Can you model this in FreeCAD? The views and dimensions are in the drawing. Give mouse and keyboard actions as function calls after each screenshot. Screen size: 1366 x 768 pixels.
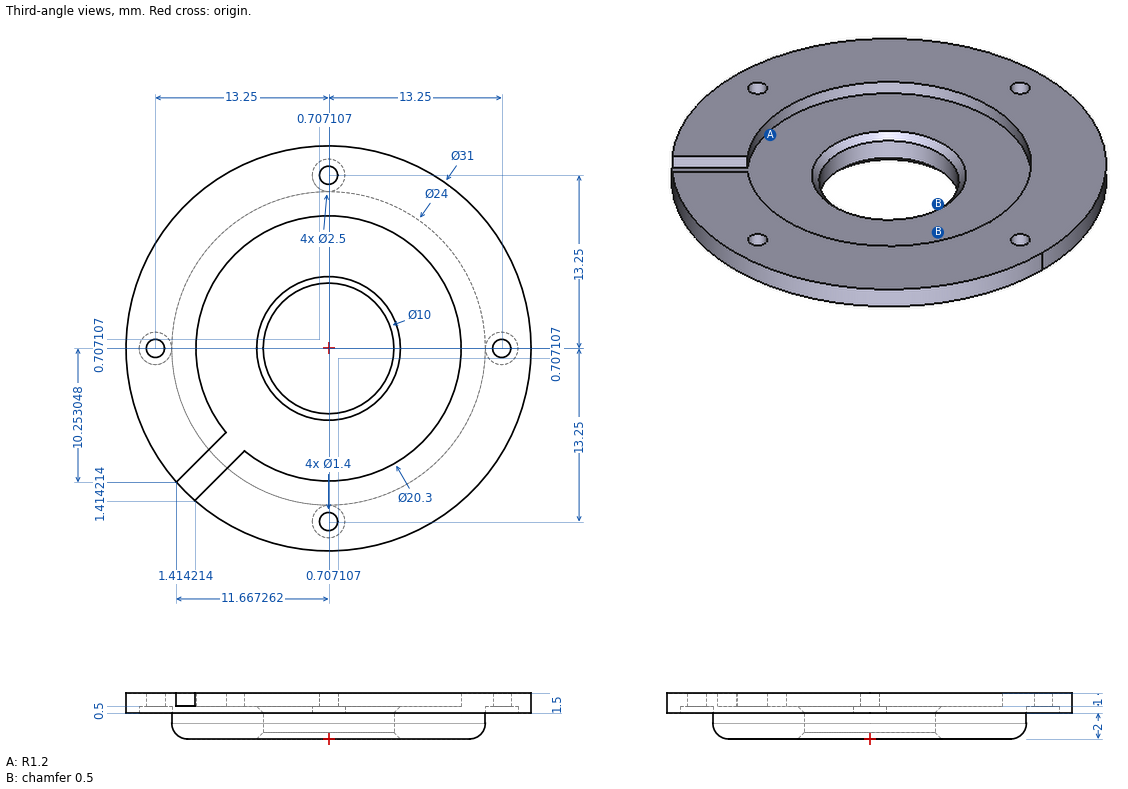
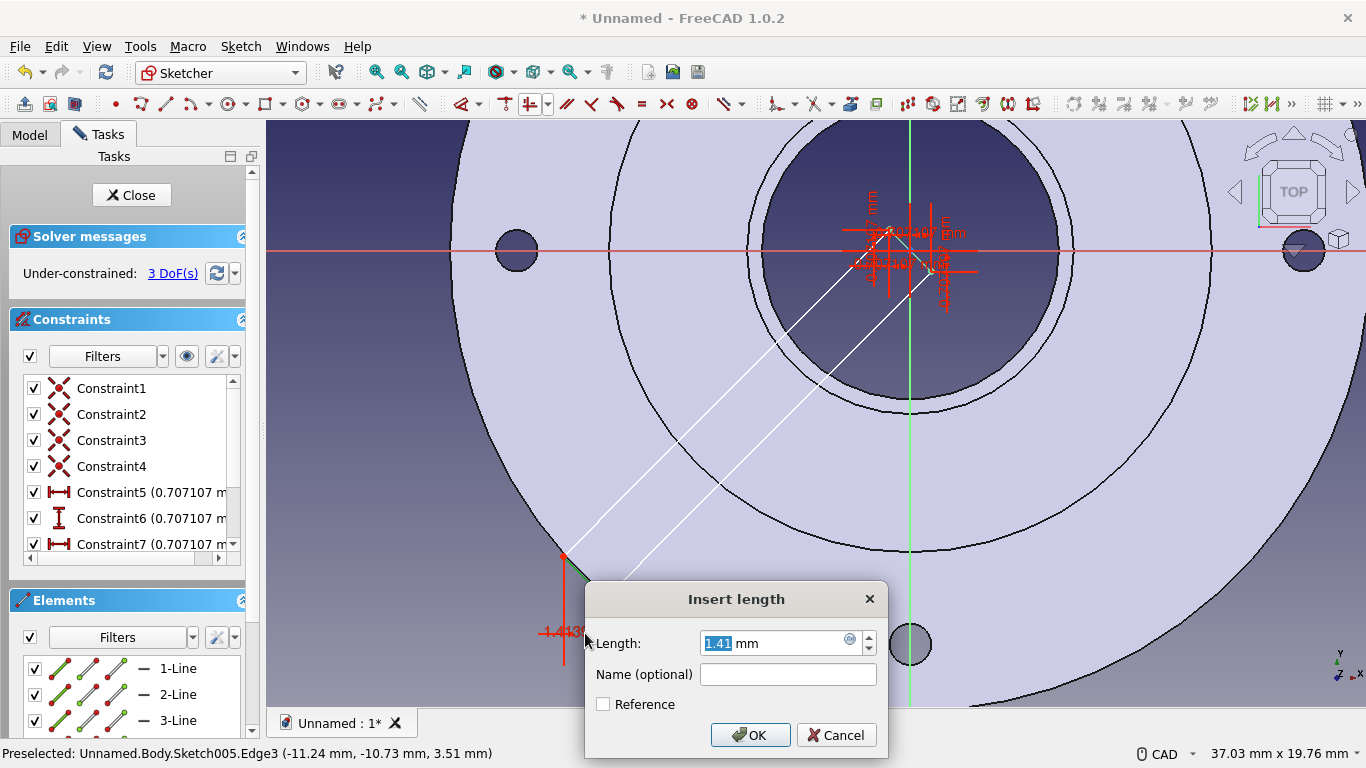
text(1.414214)
key(Return)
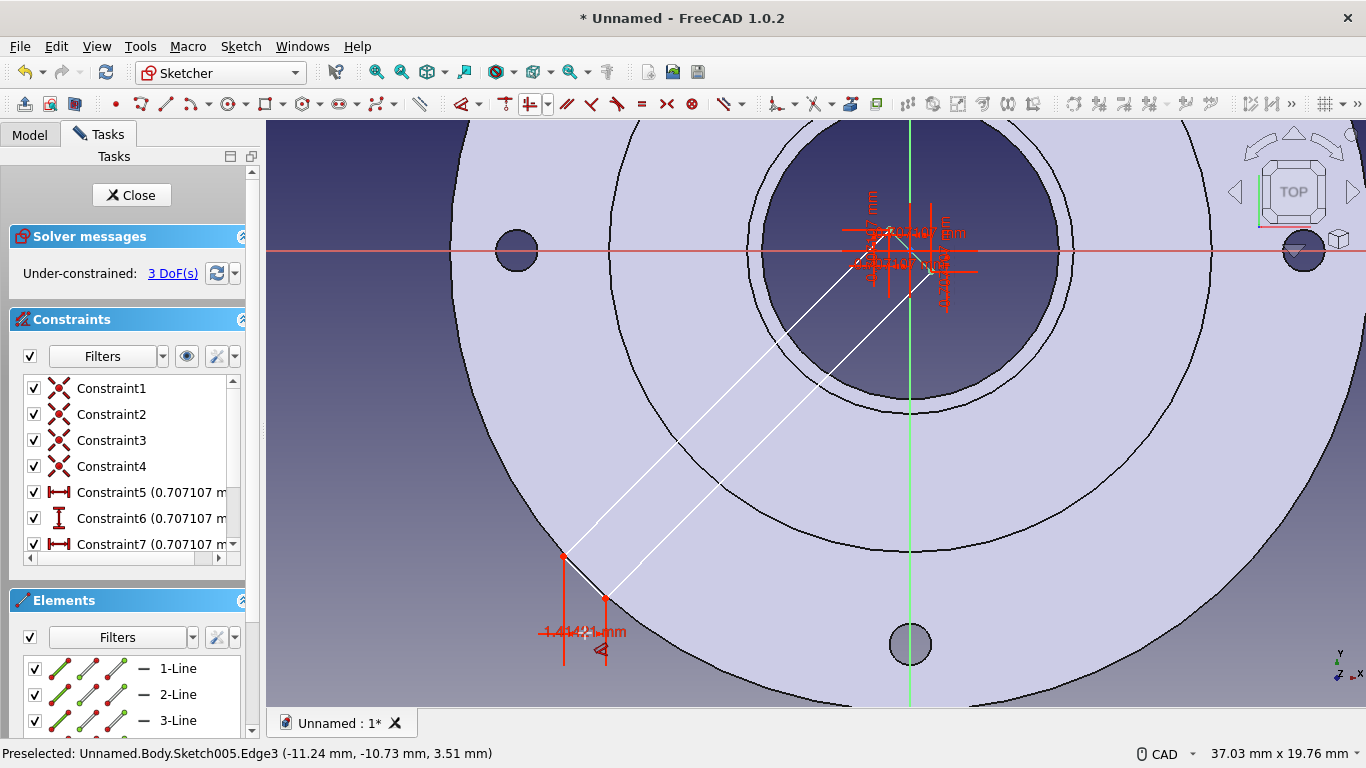
click(576, 569)
click(530, 578)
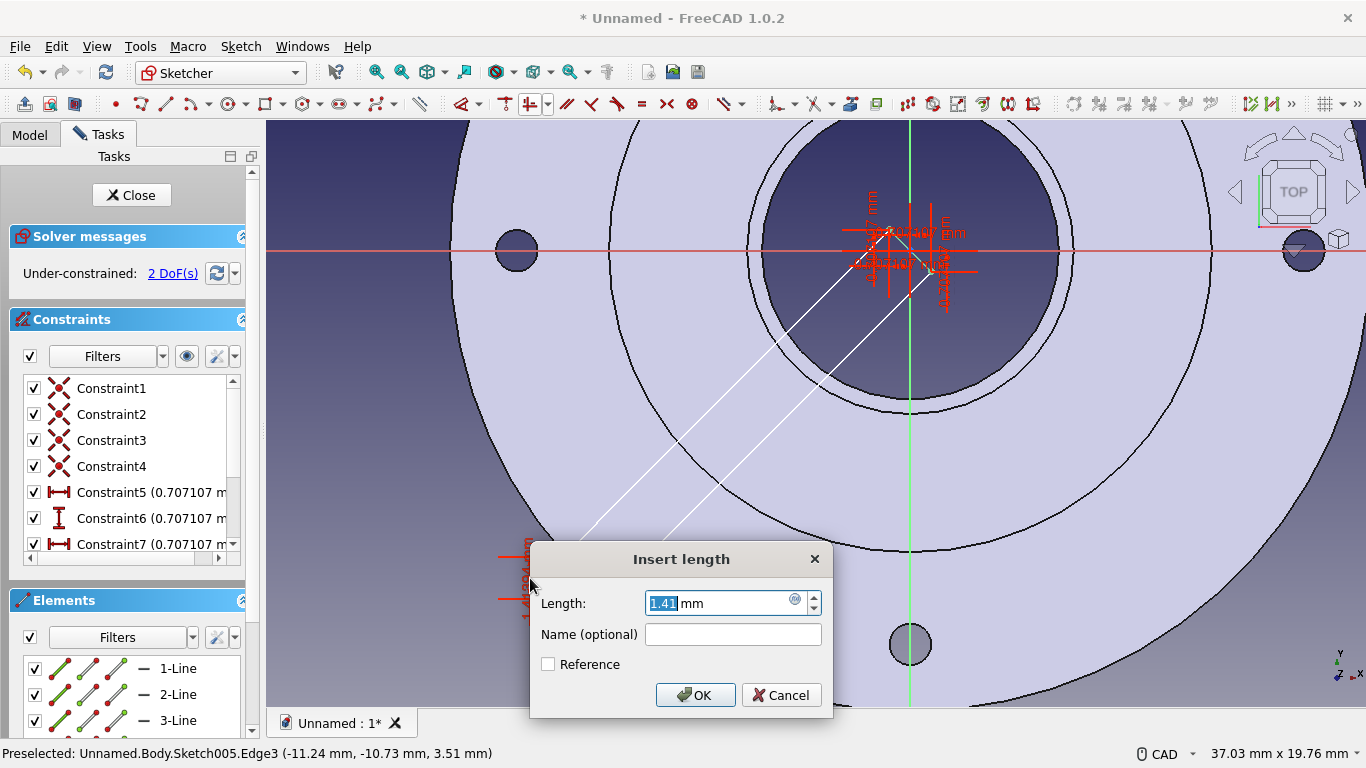
text(1.414214)
key(Return)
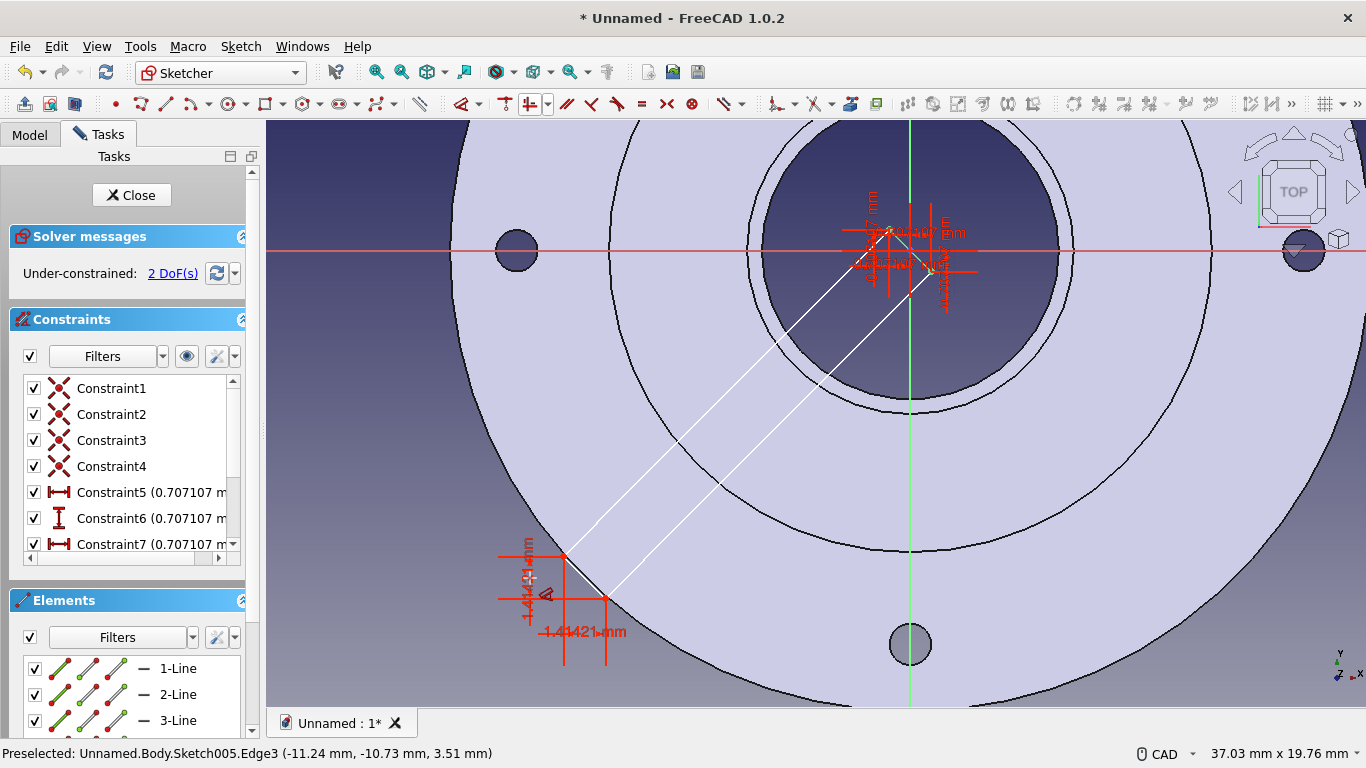
click(564, 557)
click(737, 217)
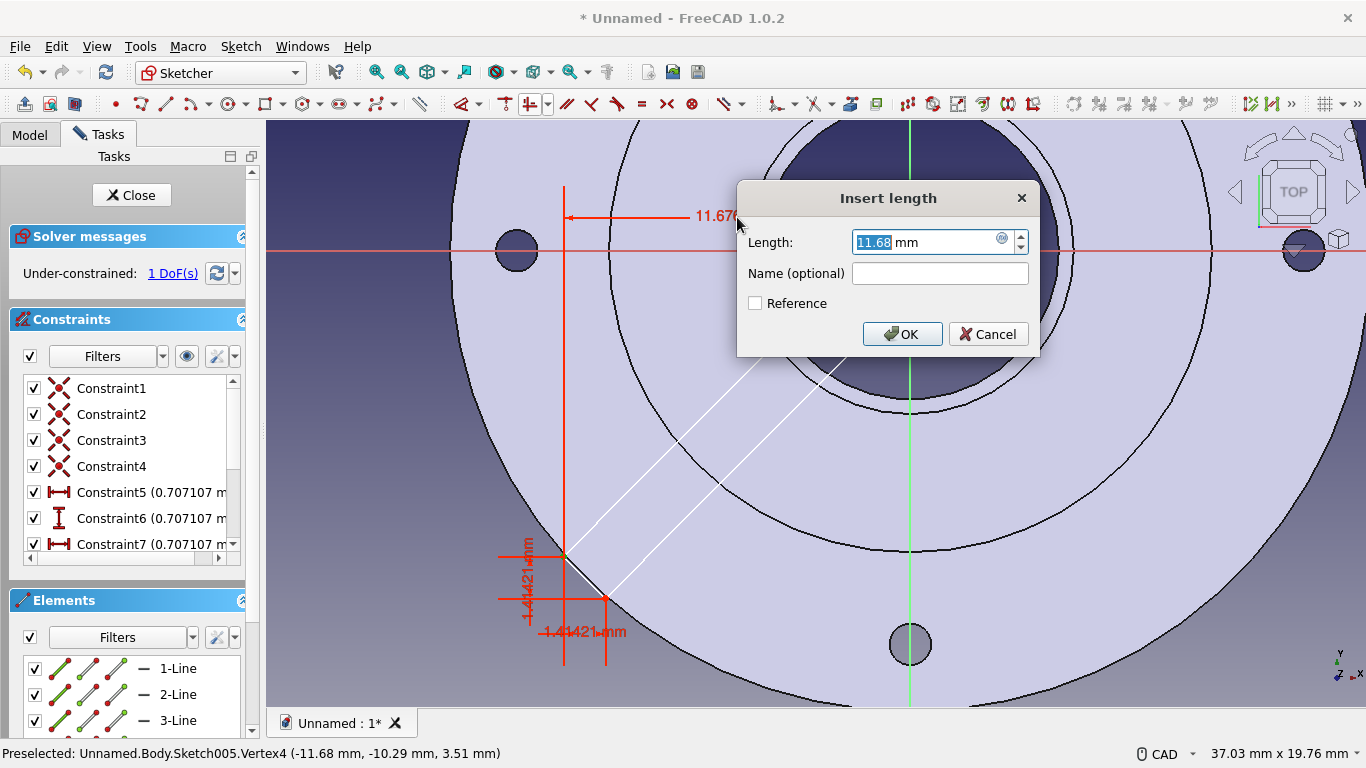
text(11.667262)
key(Return)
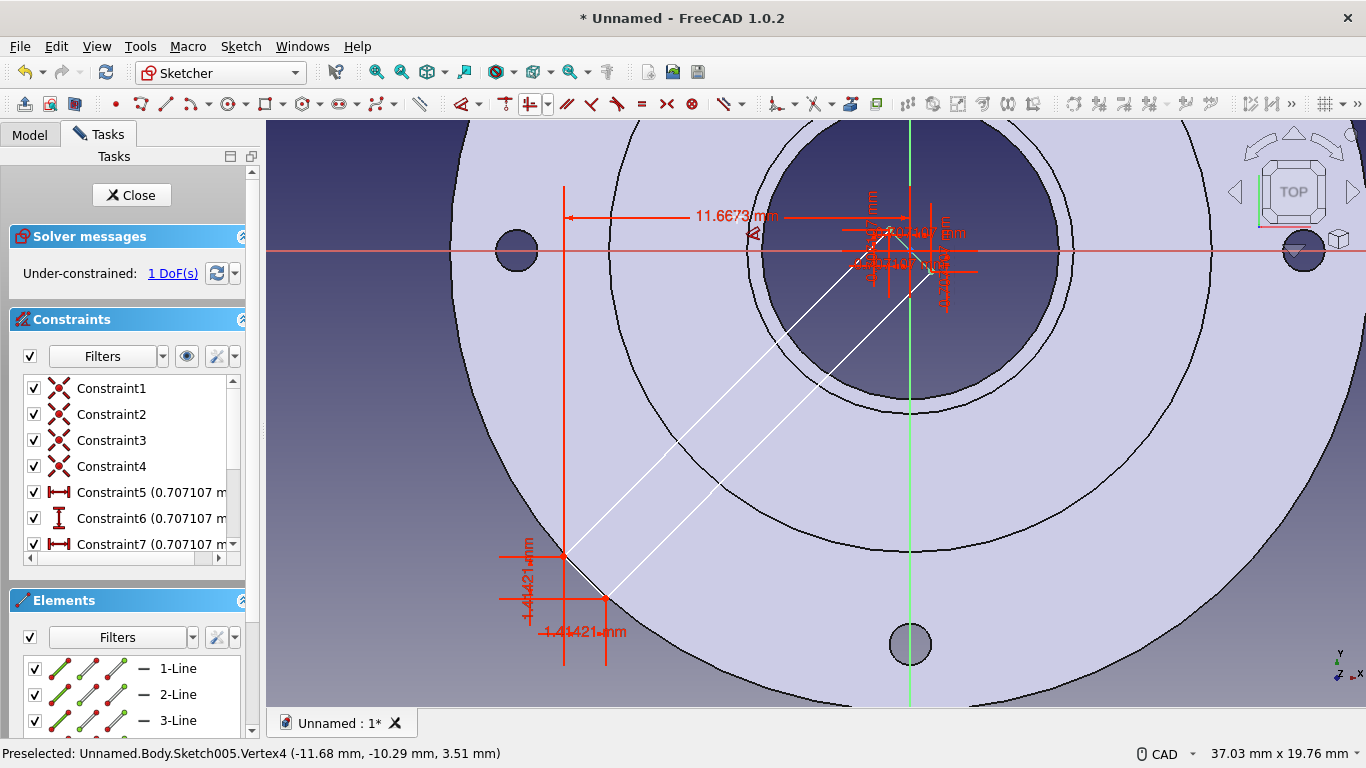
click(564, 557)
click(530, 404)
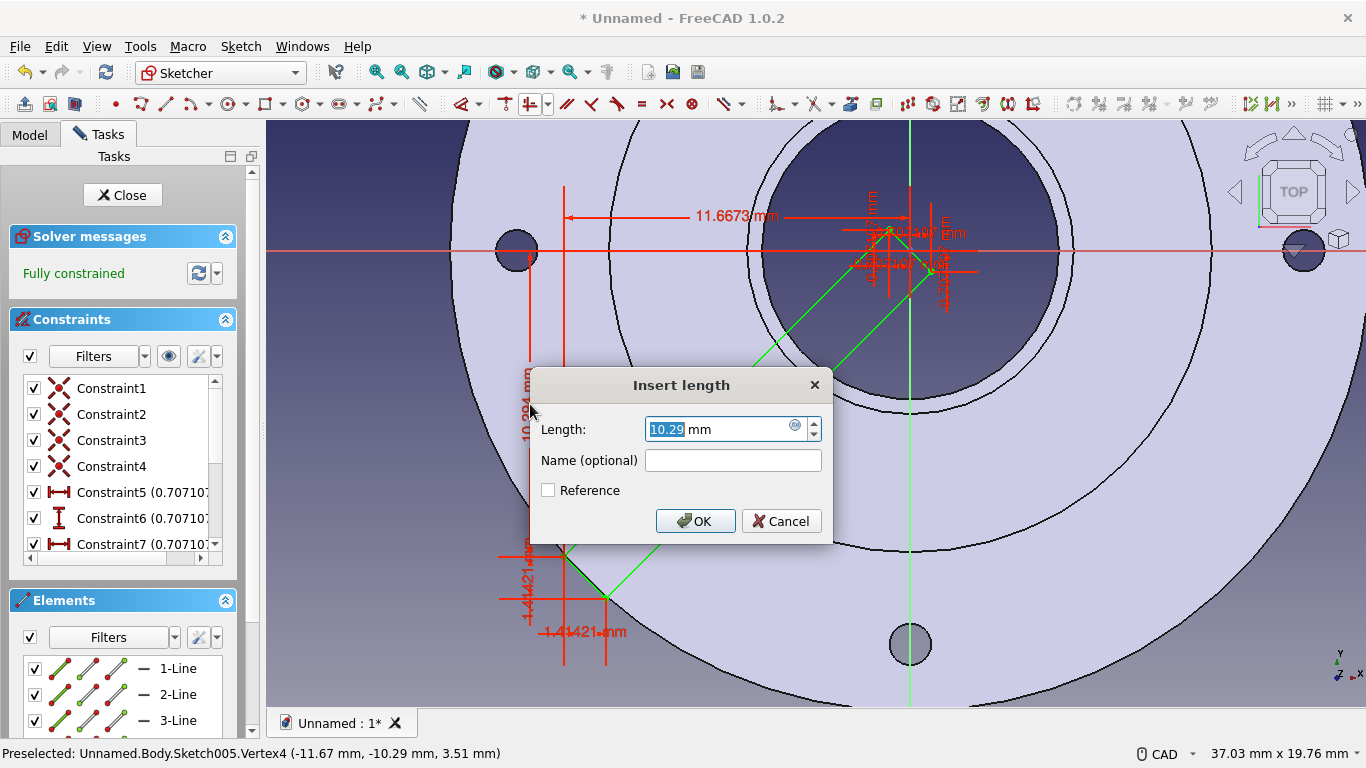
text(10.253048)
key(Return)
key(Escape)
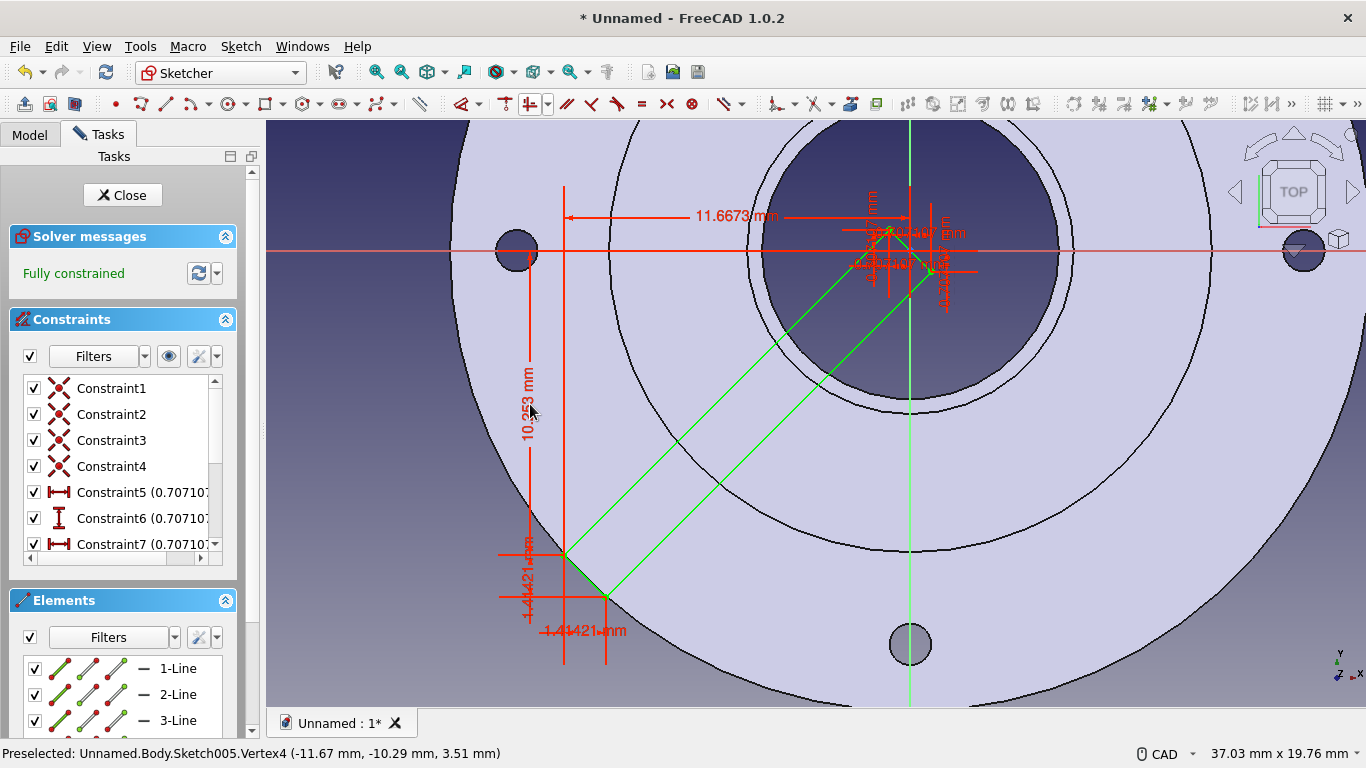
click(123, 195)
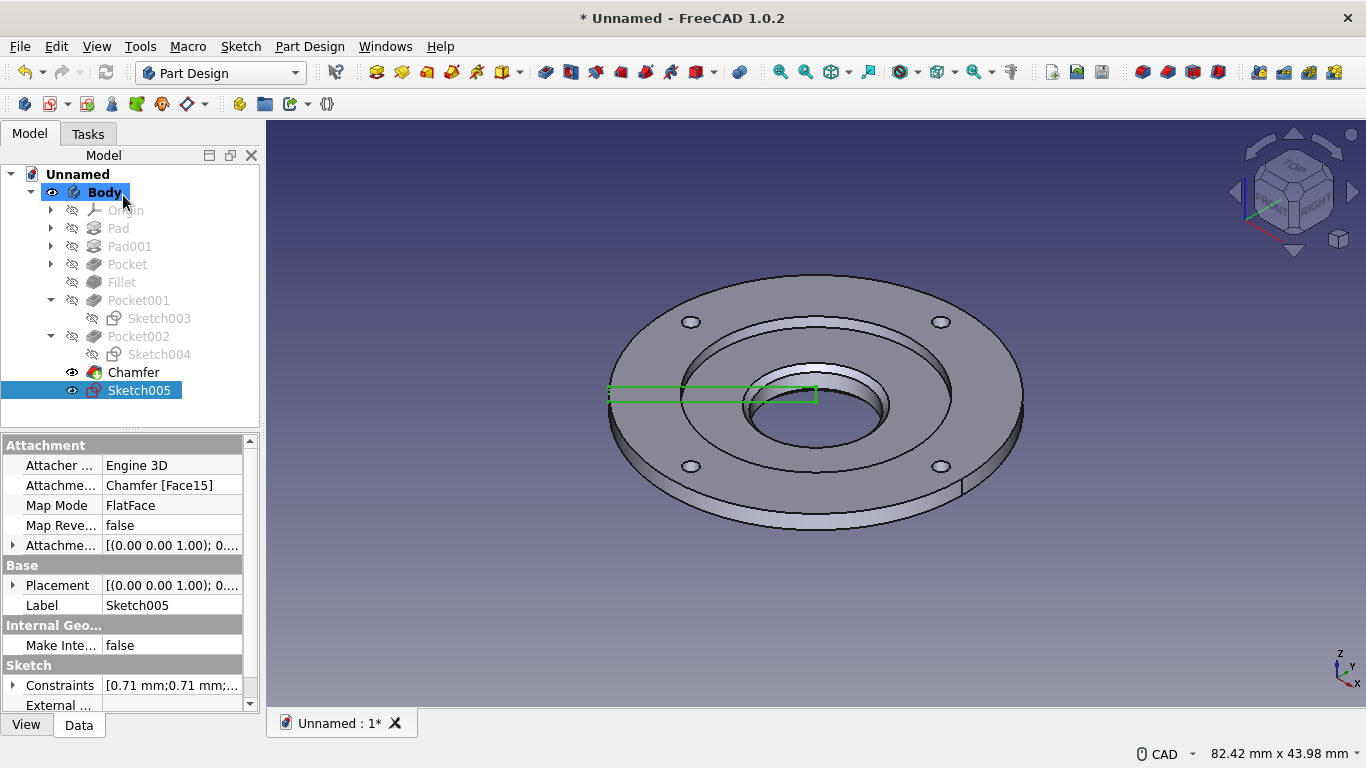
click(546, 72)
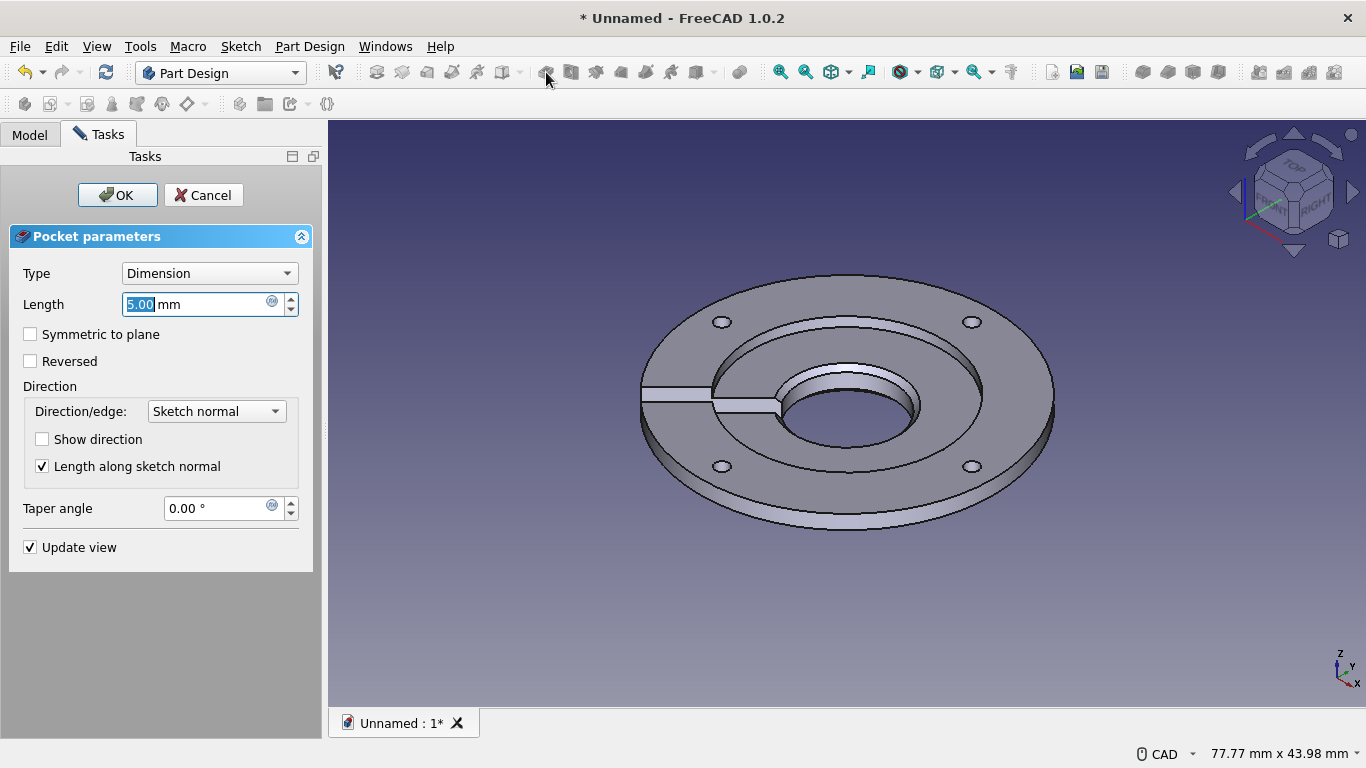
text(1)
key(Tab)